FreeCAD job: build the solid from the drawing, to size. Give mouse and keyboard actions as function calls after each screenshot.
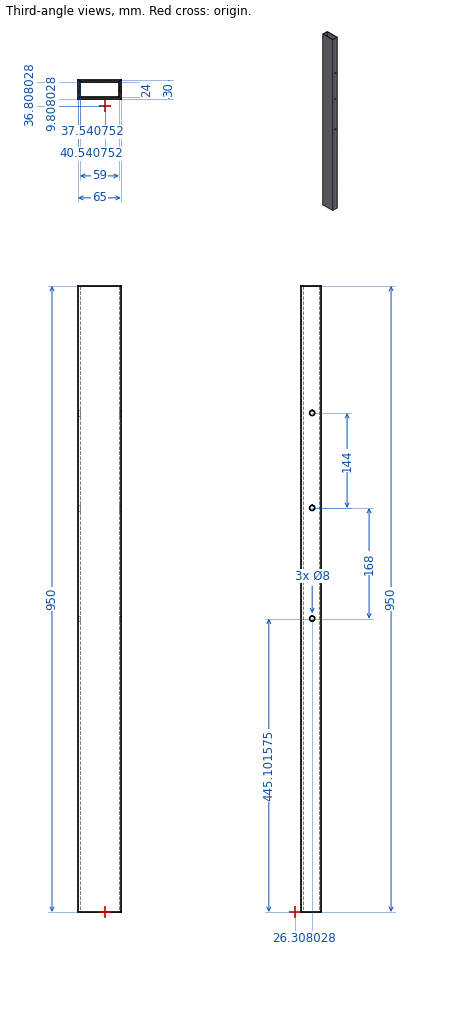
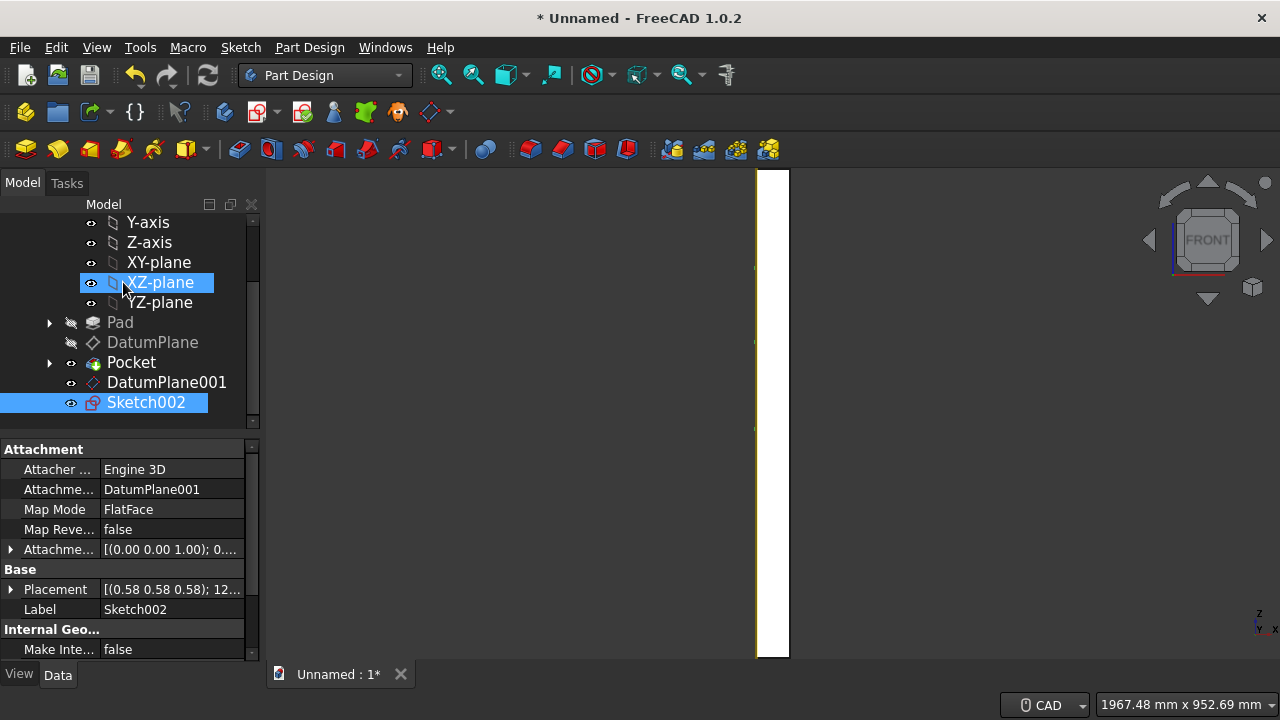
click(240, 150)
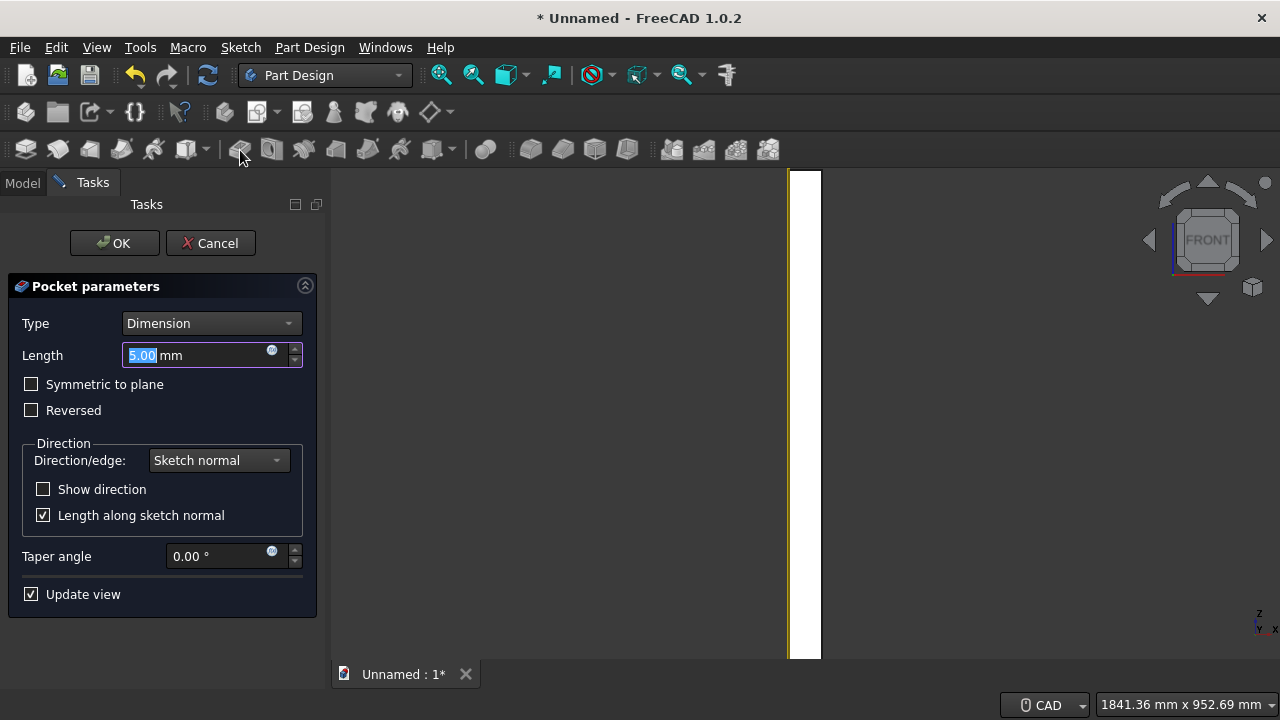
click(212, 324)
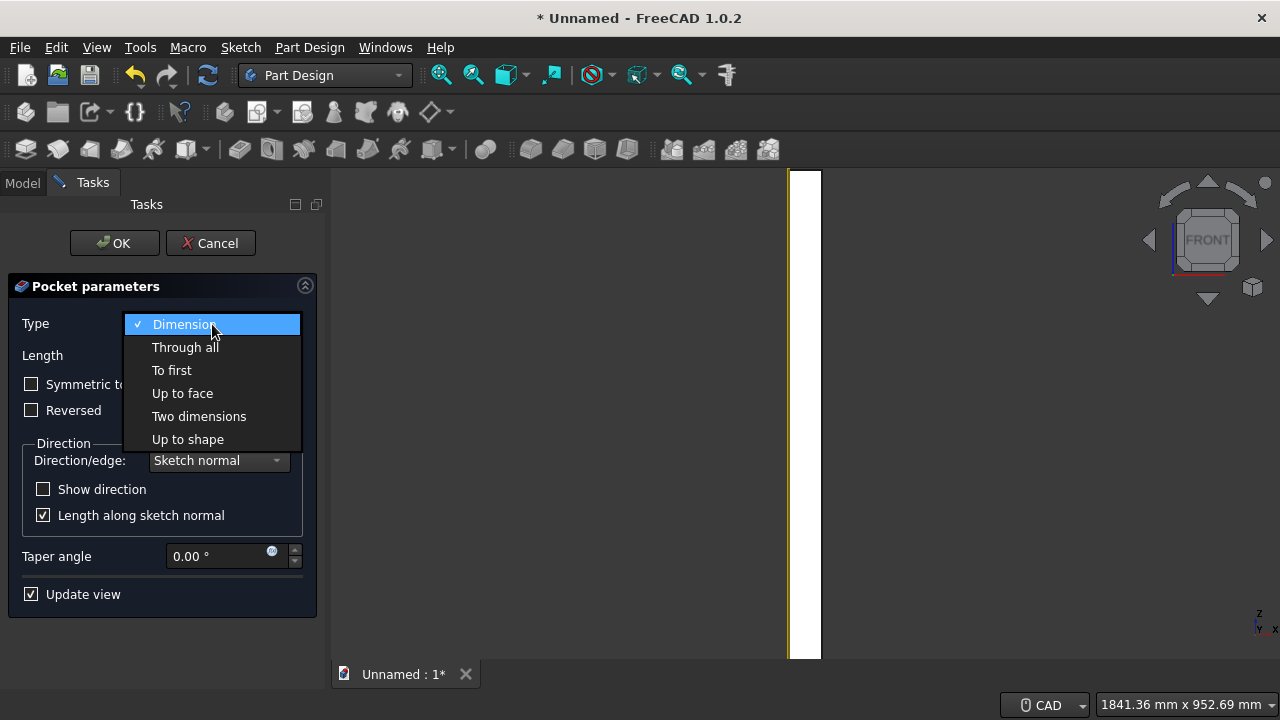
click(212, 348)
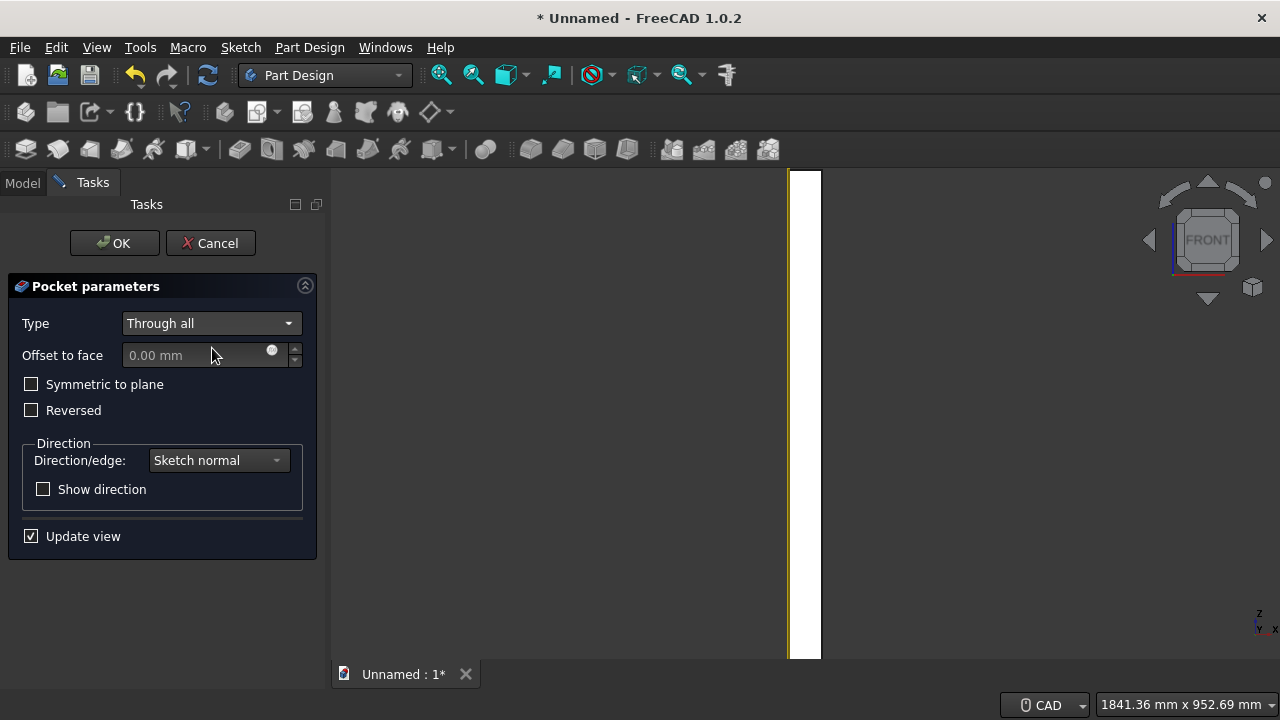
click(30, 410)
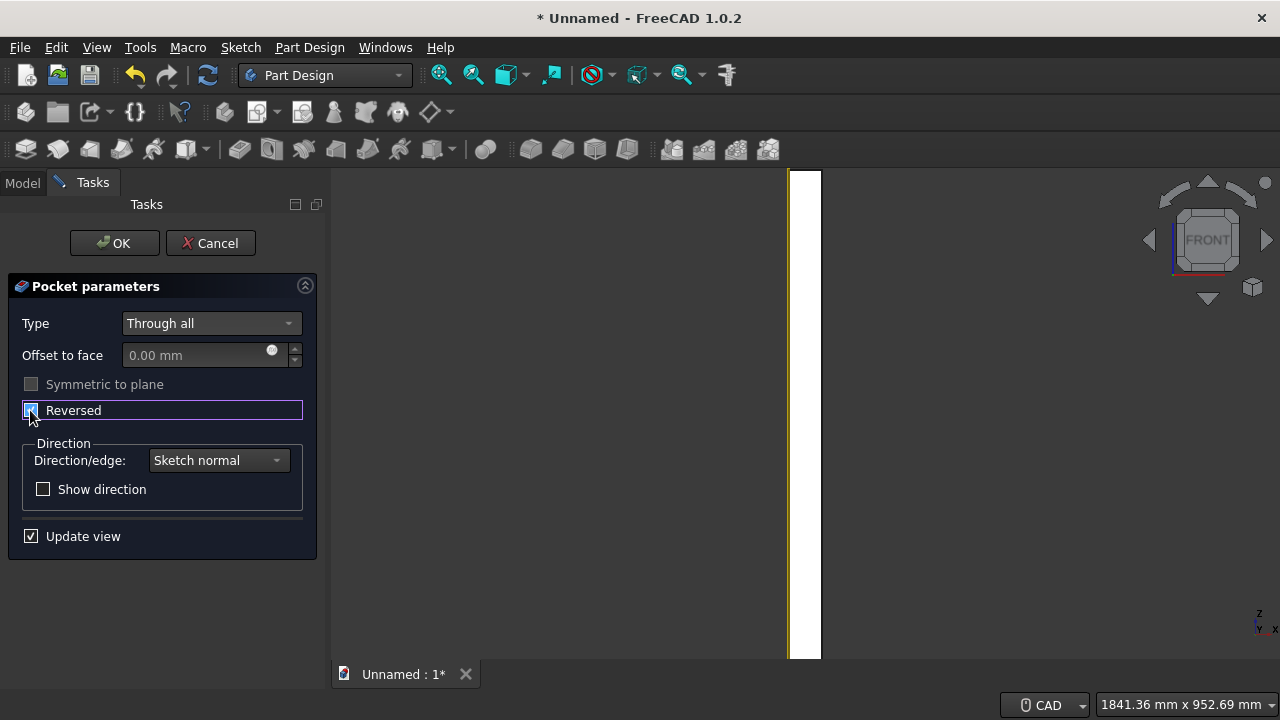
click(115, 243)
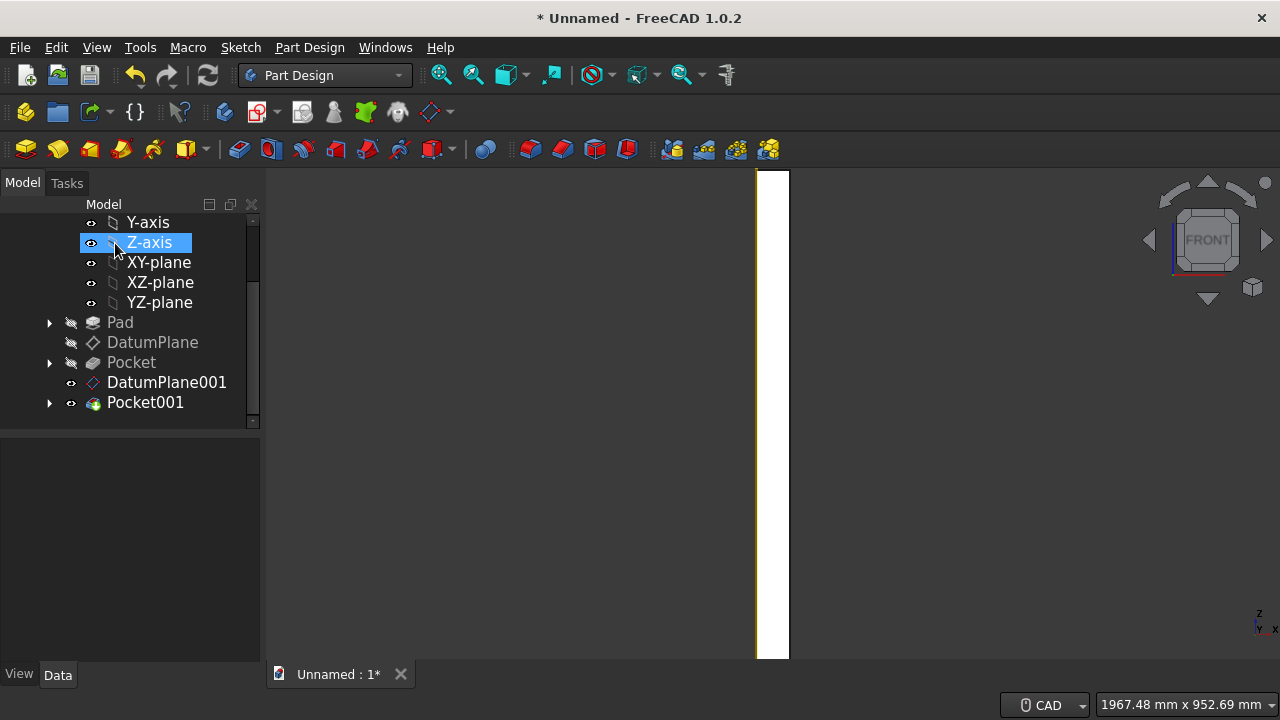
click(116, 383)
key(space)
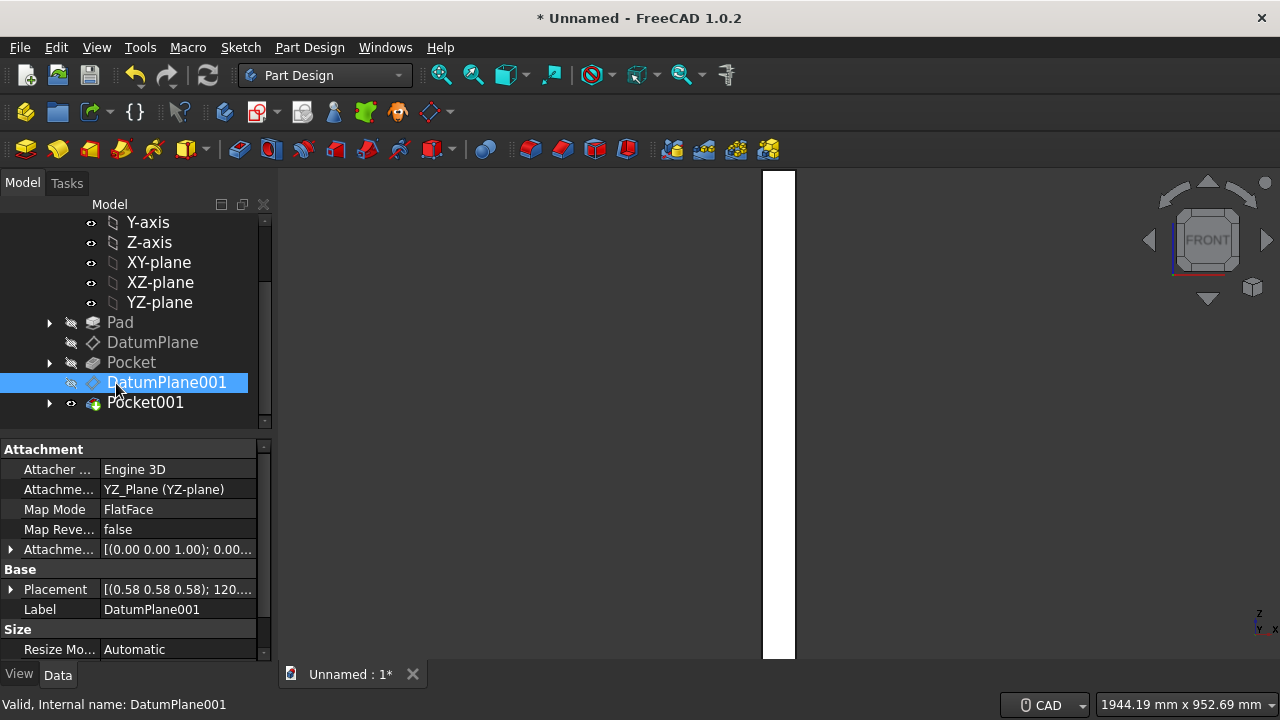
key(0)